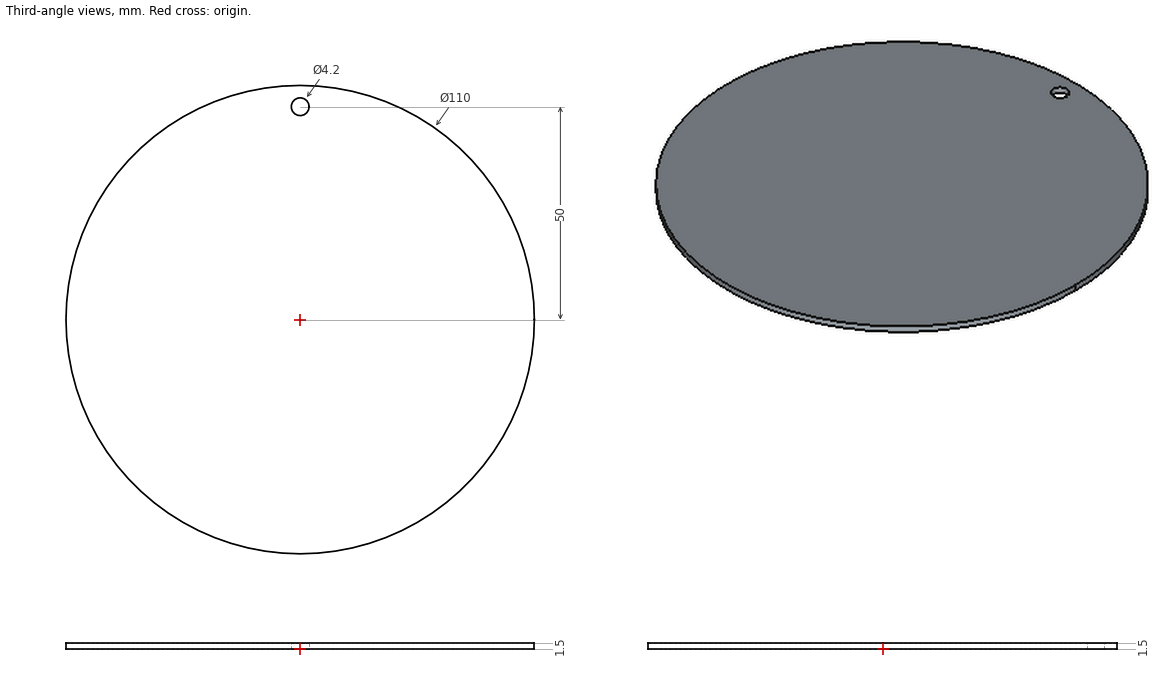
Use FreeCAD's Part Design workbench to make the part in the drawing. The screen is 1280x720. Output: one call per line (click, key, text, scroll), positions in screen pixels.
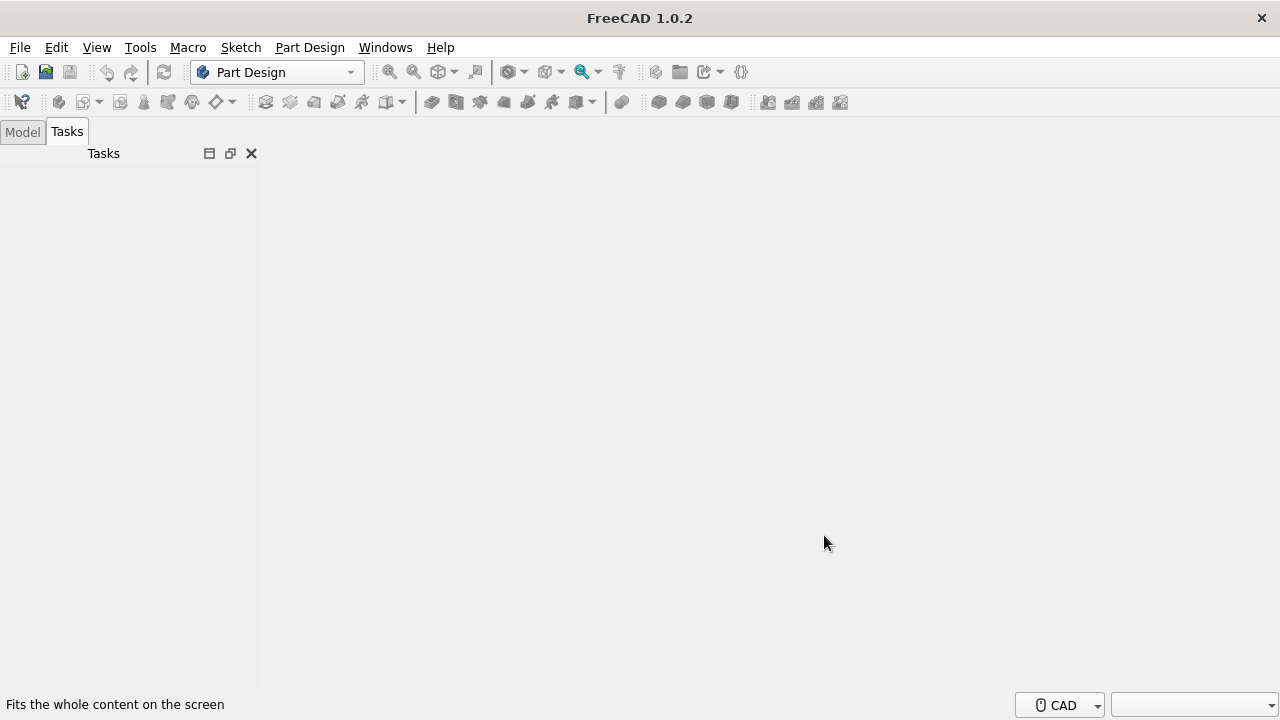
click(22, 72)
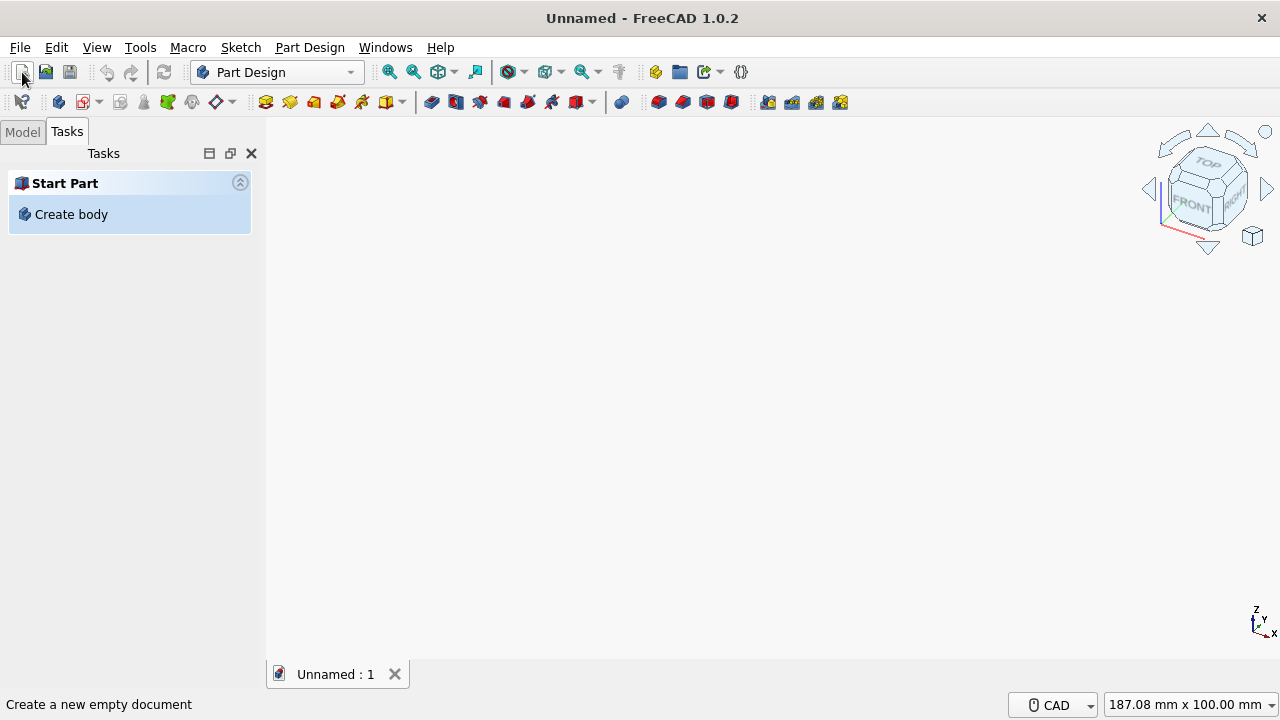
click(84, 102)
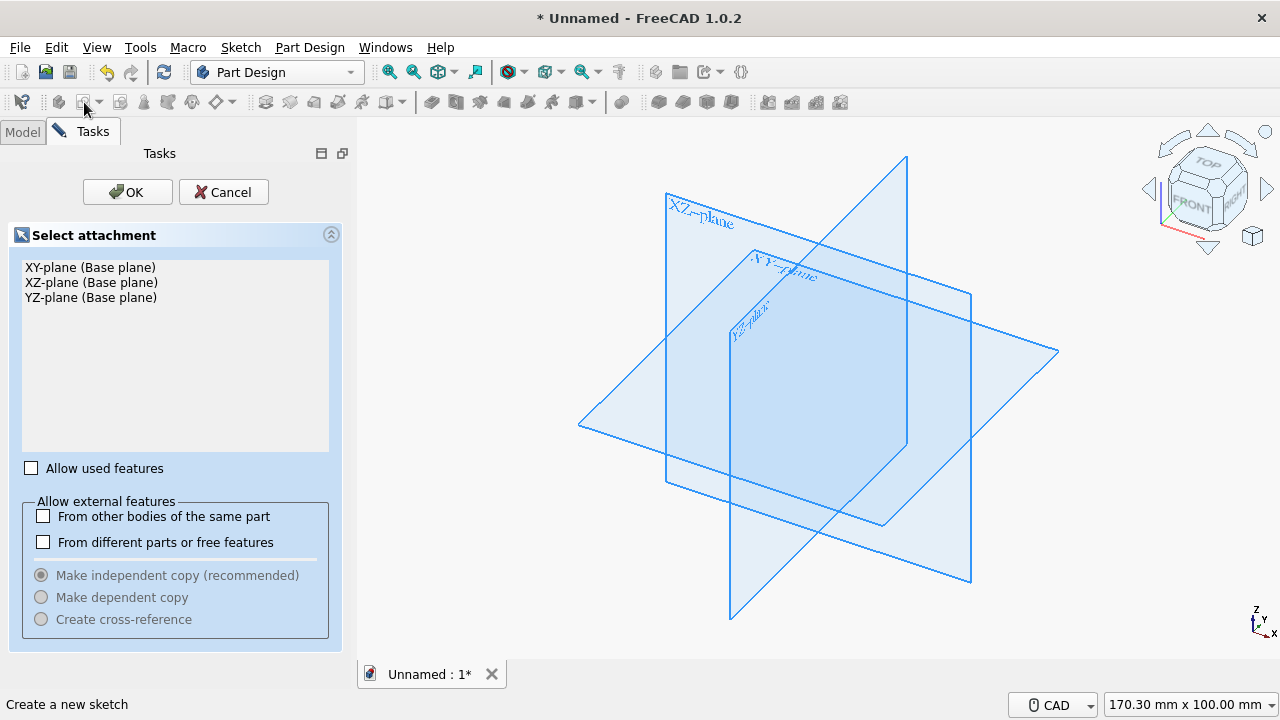
click(82, 268)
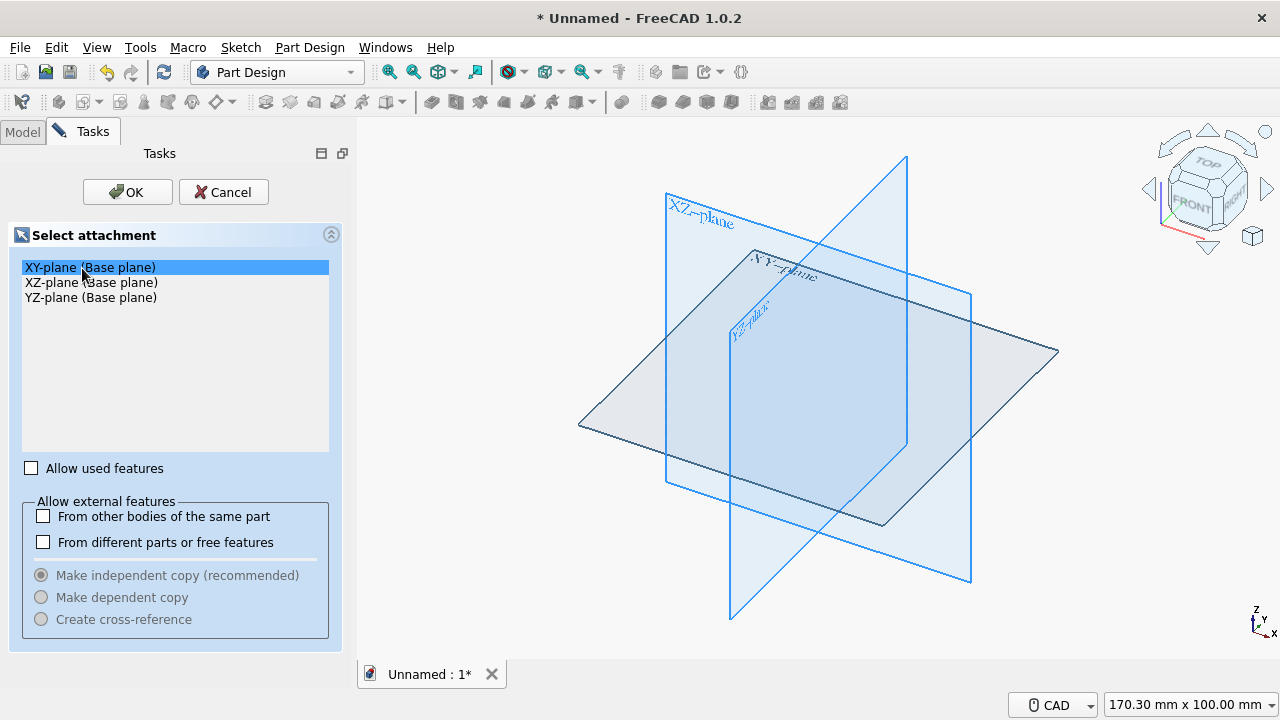
click(128, 192)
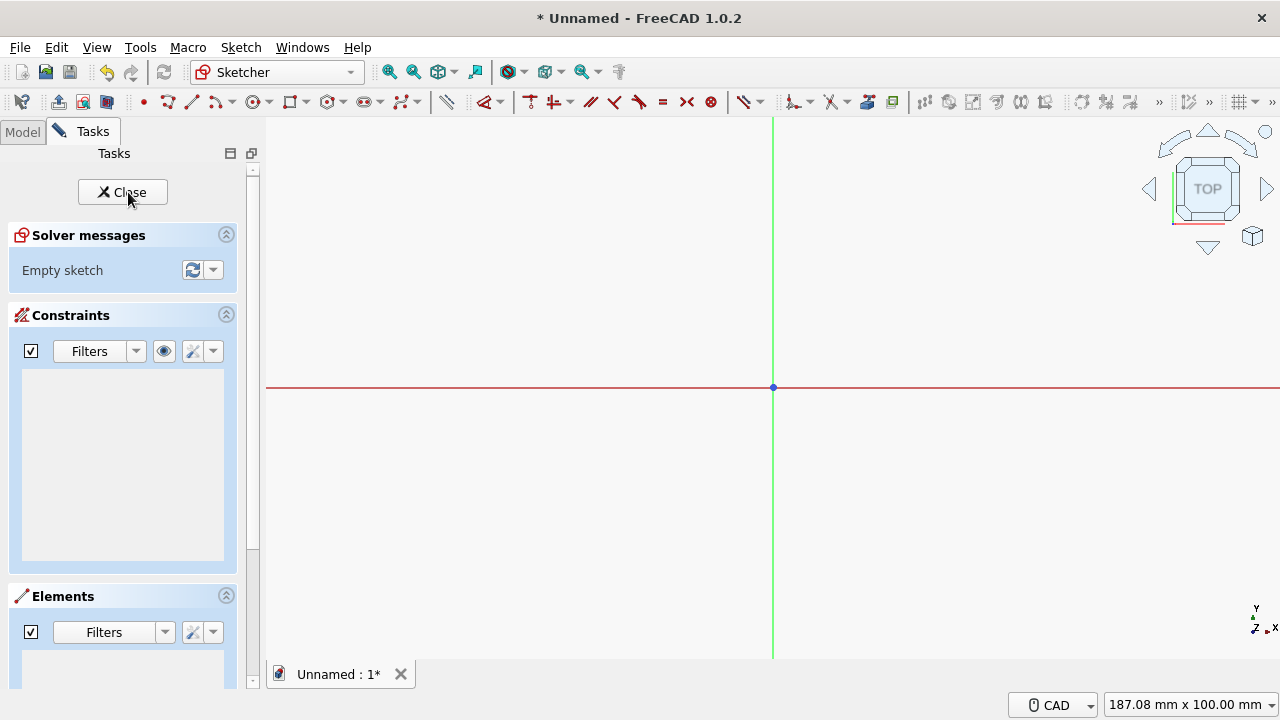
scroll(621, 388, down, 3)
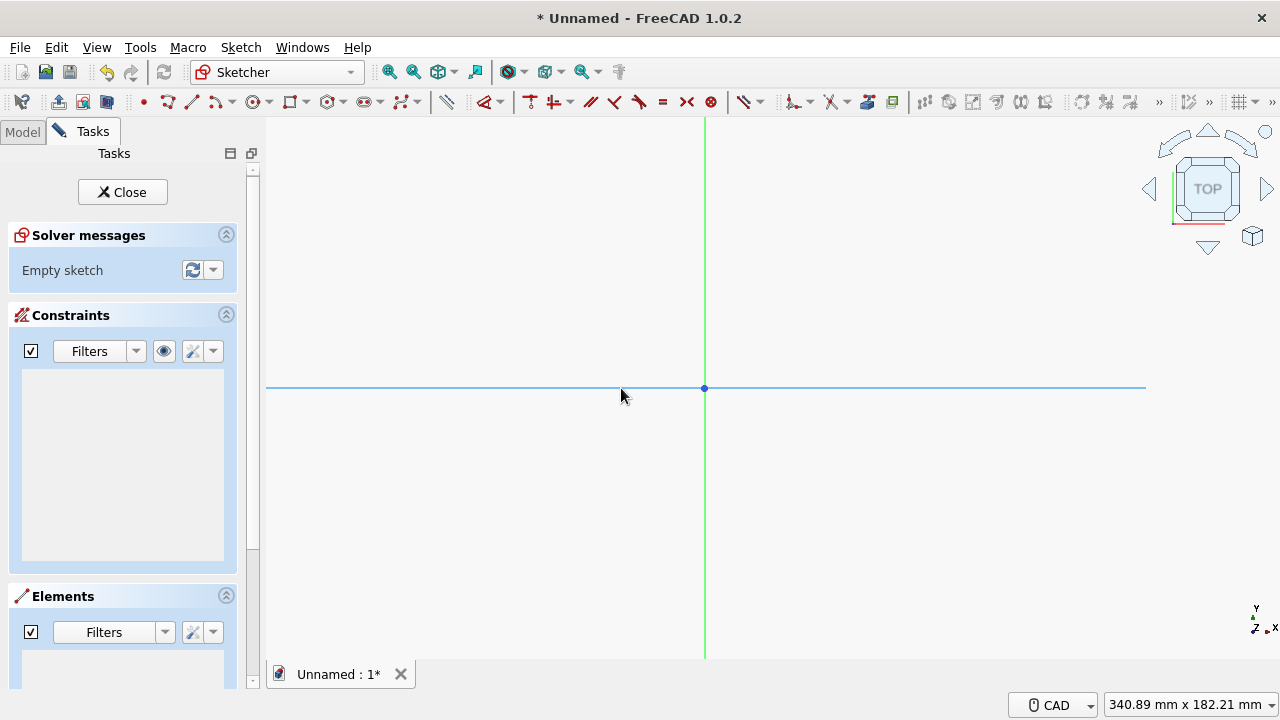
click(254, 102)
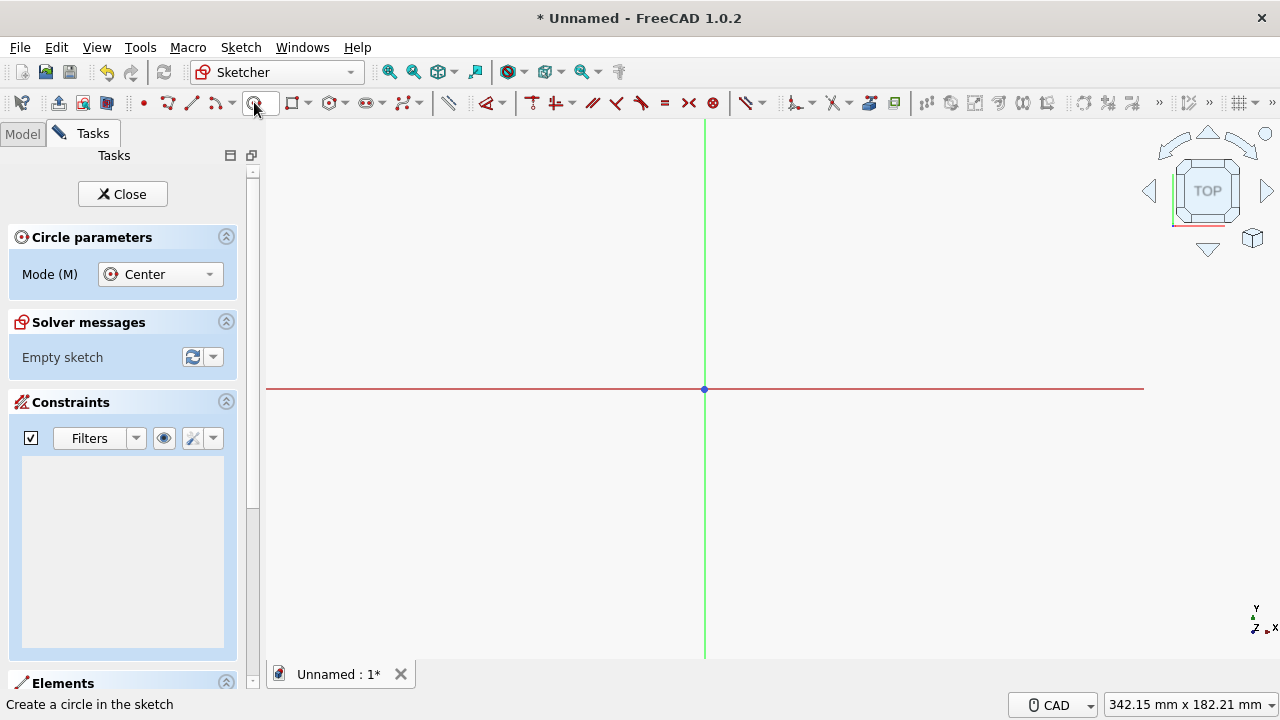
click(705, 389)
click(820, 274)
key(Escape)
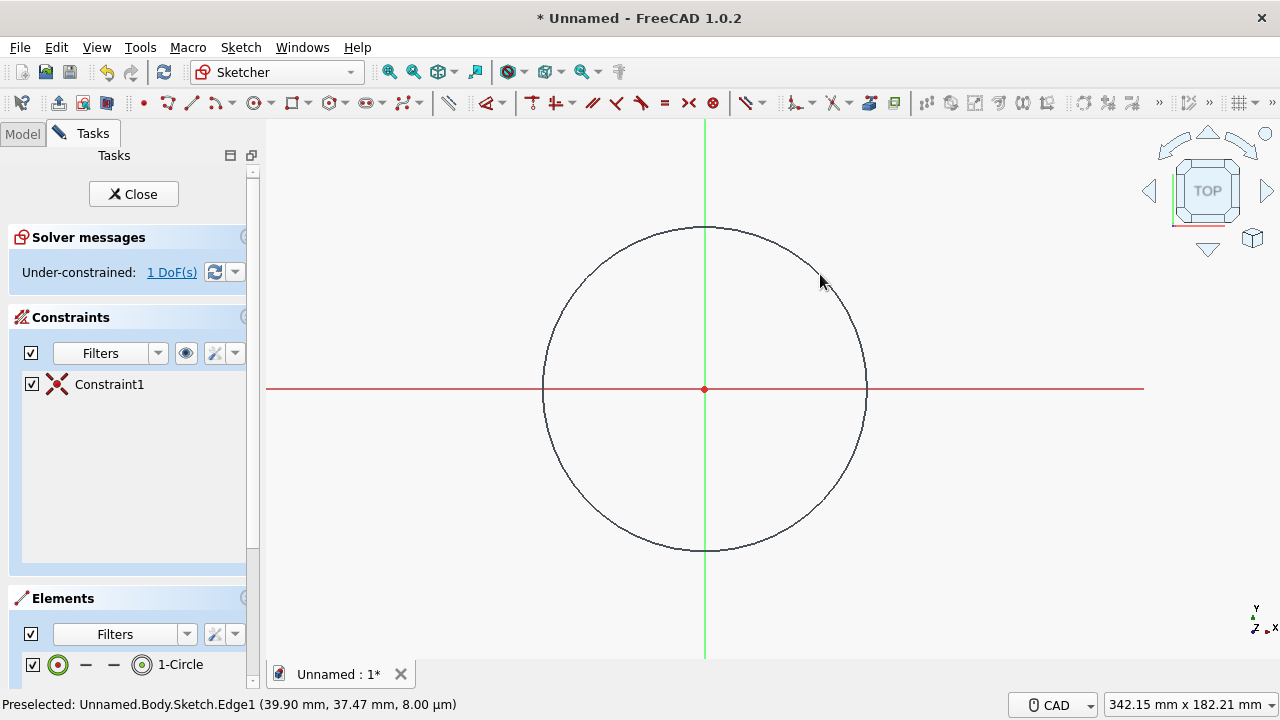
click(486, 104)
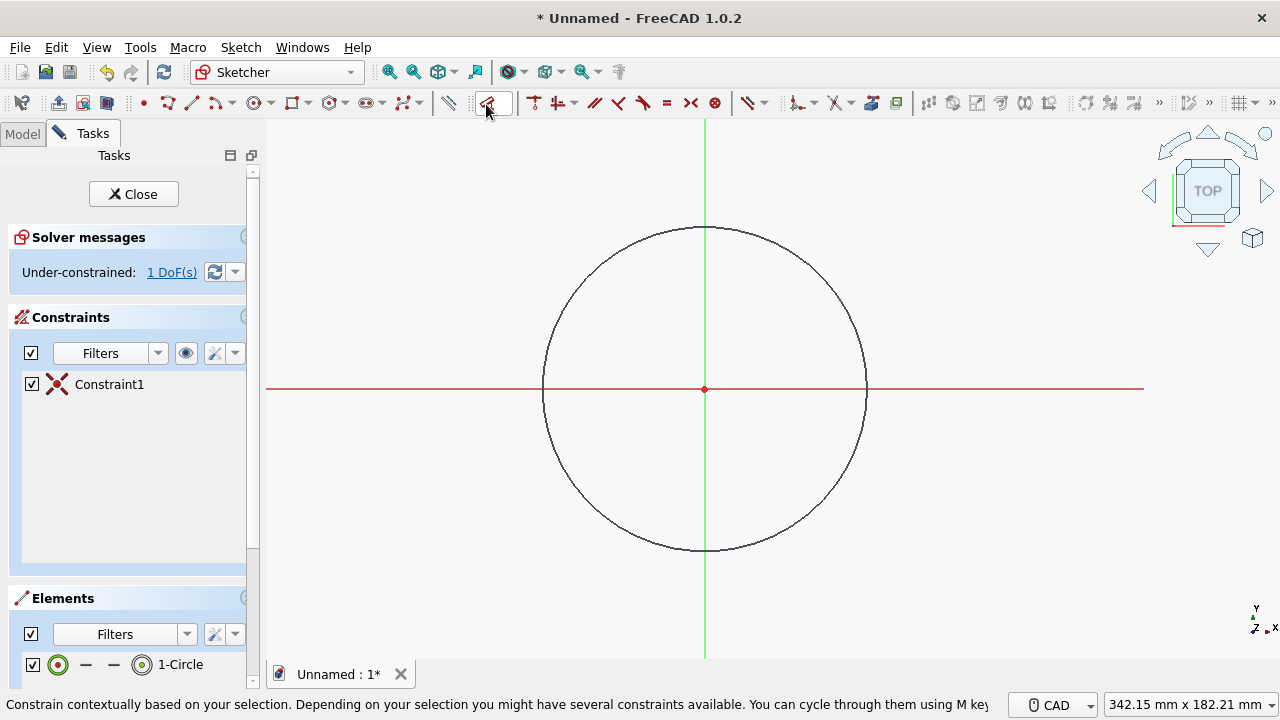
click(819, 274)
click(842, 251)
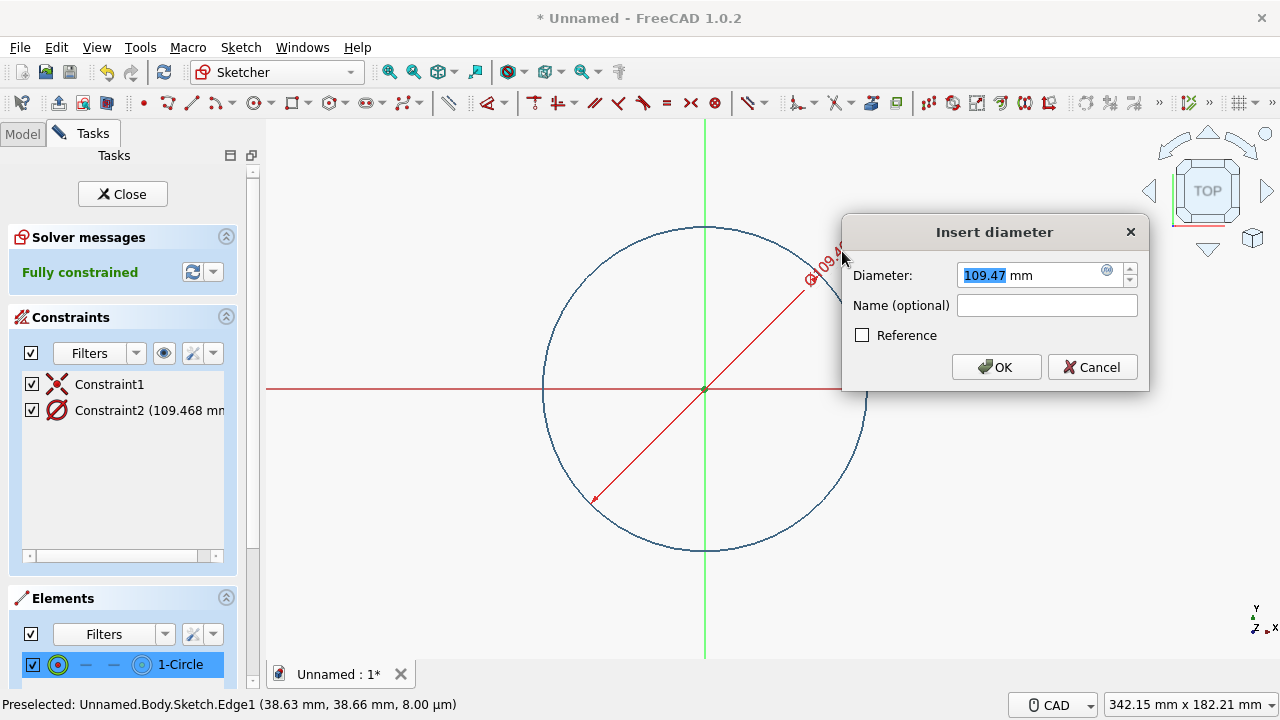
text(110)
key(Return)
key(Escape)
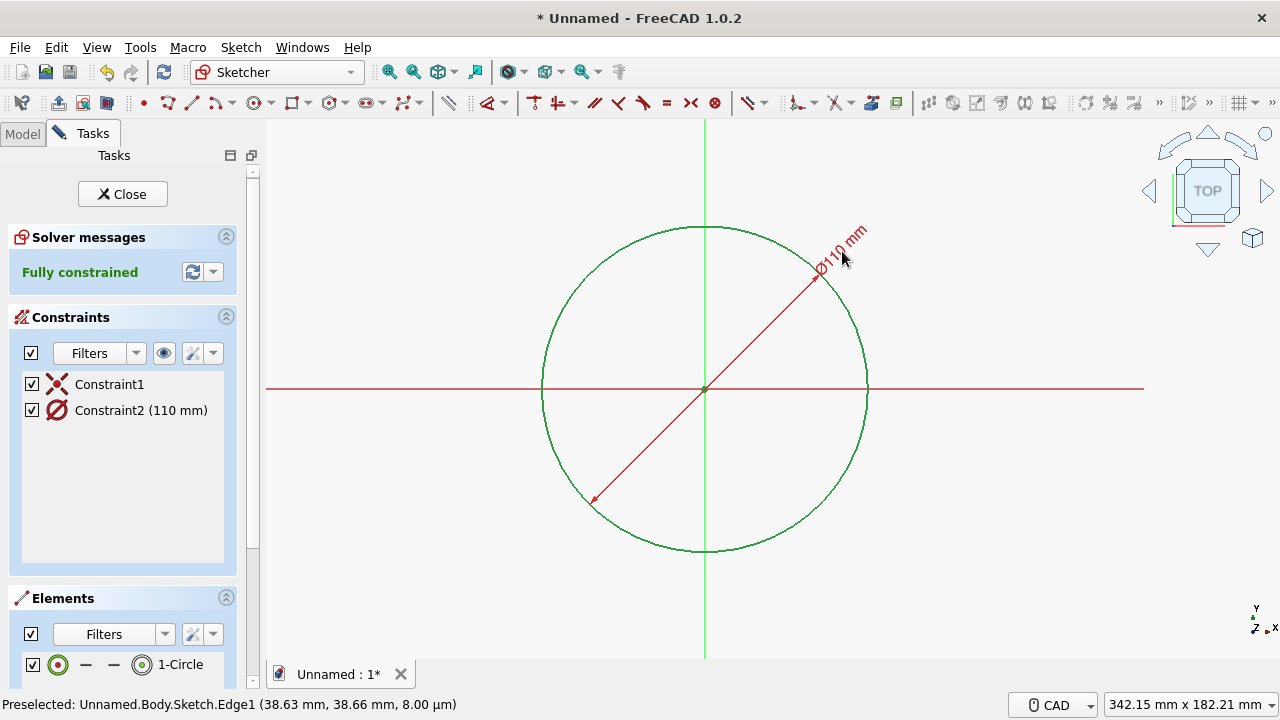
click(123, 194)